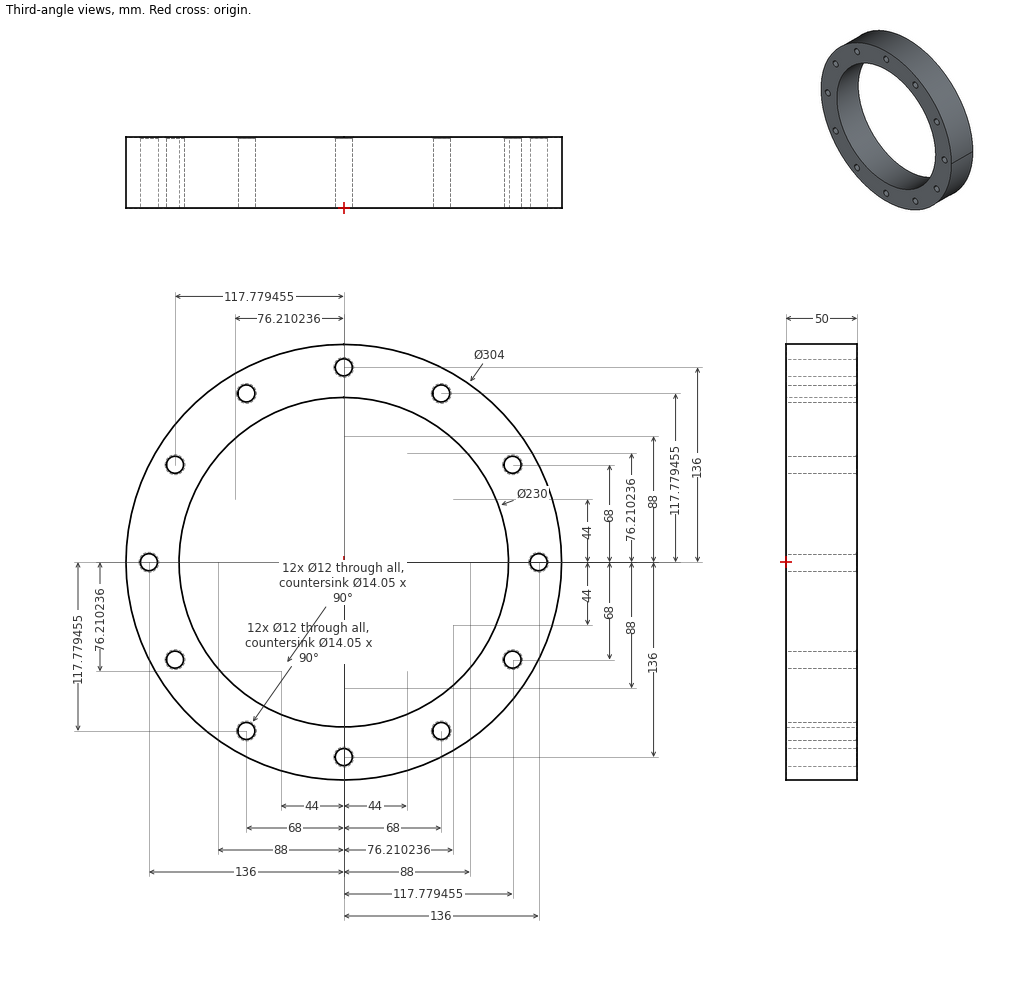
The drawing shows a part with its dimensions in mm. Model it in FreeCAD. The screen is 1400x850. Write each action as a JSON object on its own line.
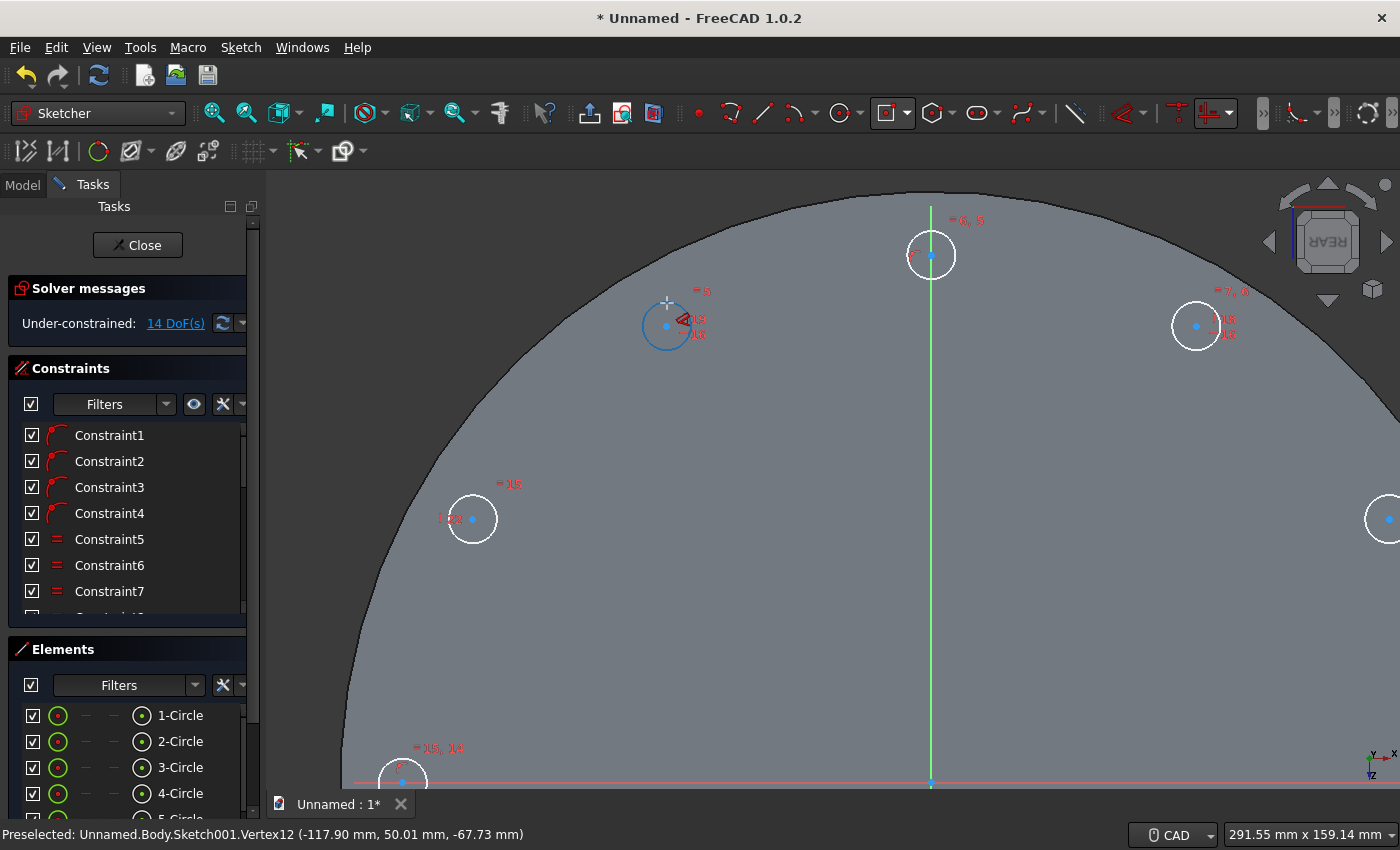
{"action": "left_click", "coordinate": [668, 302]}
{"action": "left_click", "coordinate": [669, 270]}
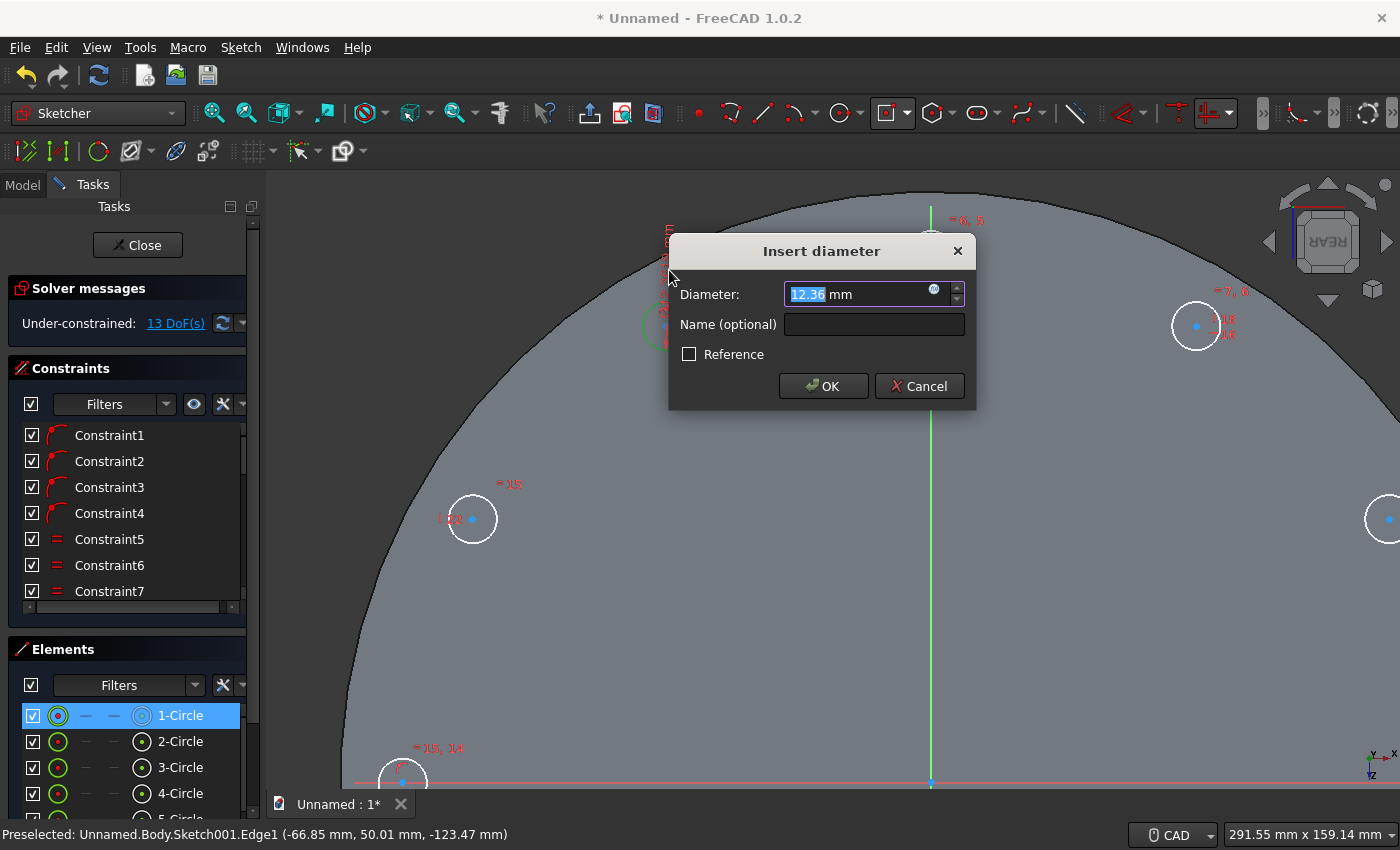
{"action": "type", "text": "12"}
{"action": "key", "text": "Return"}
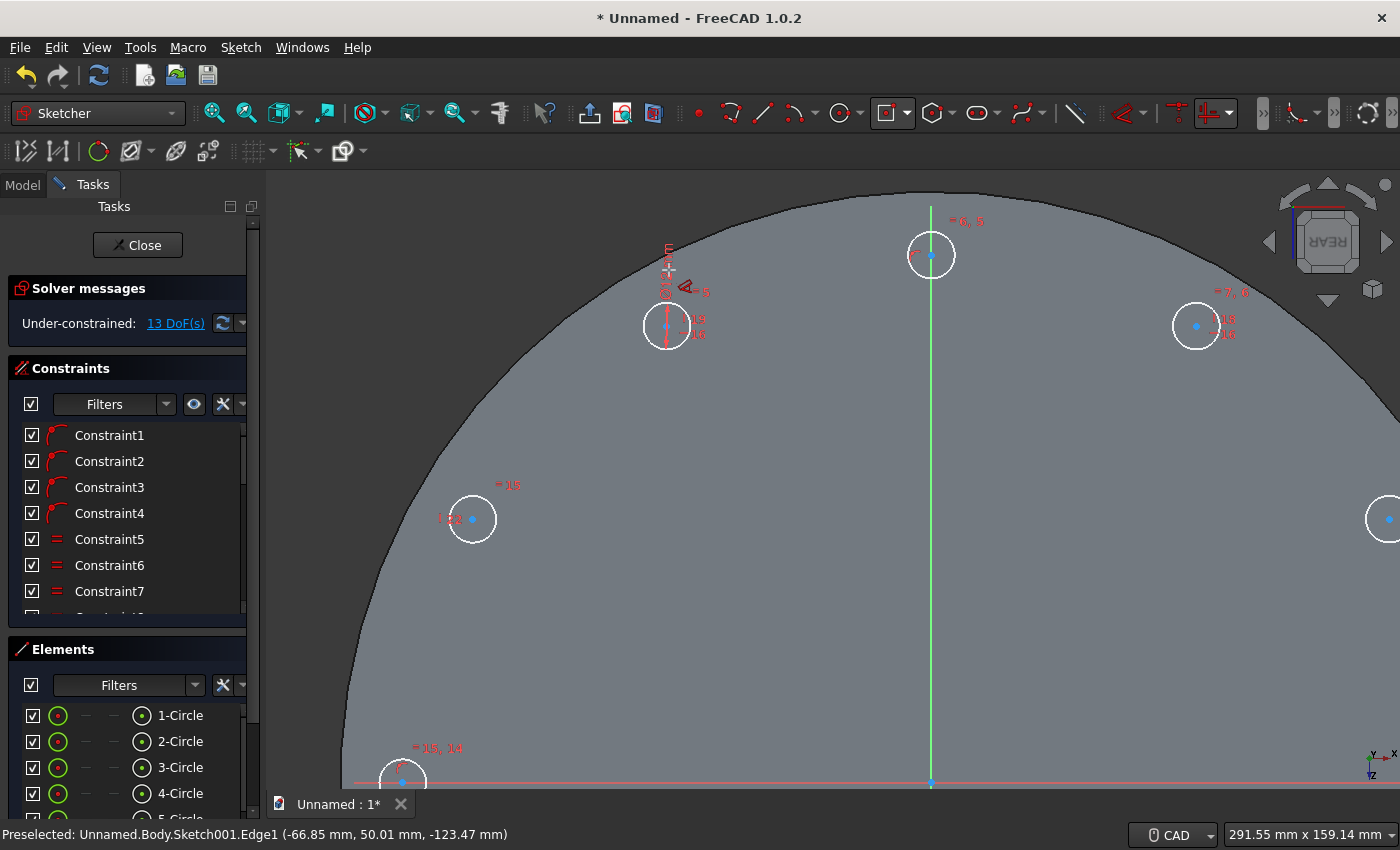
{"action": "left_click", "coordinate": [667, 326]}
{"action": "left_click", "coordinate": [799, 292]}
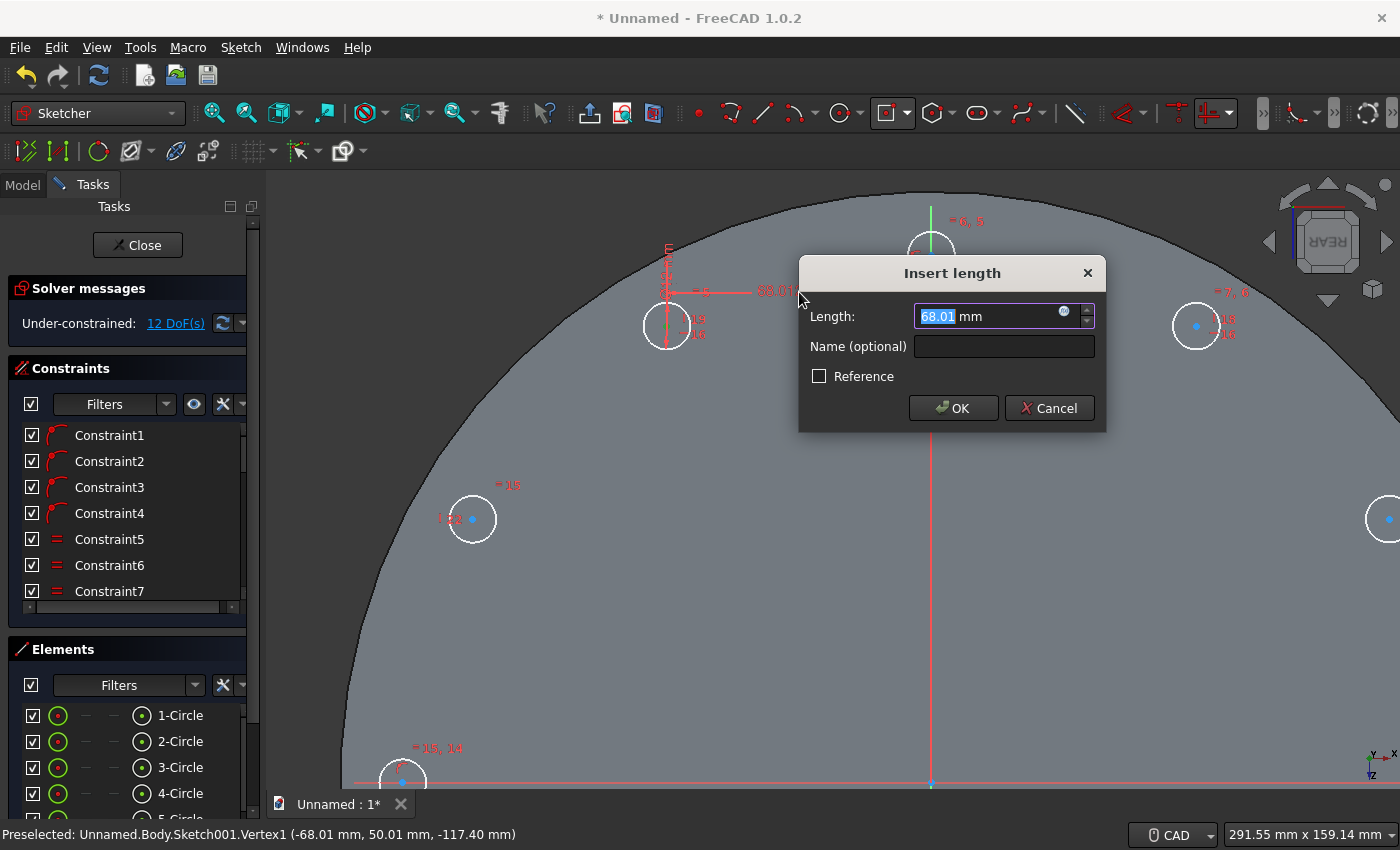
{"action": "type", "text": "68"}
{"action": "key", "text": "Return"}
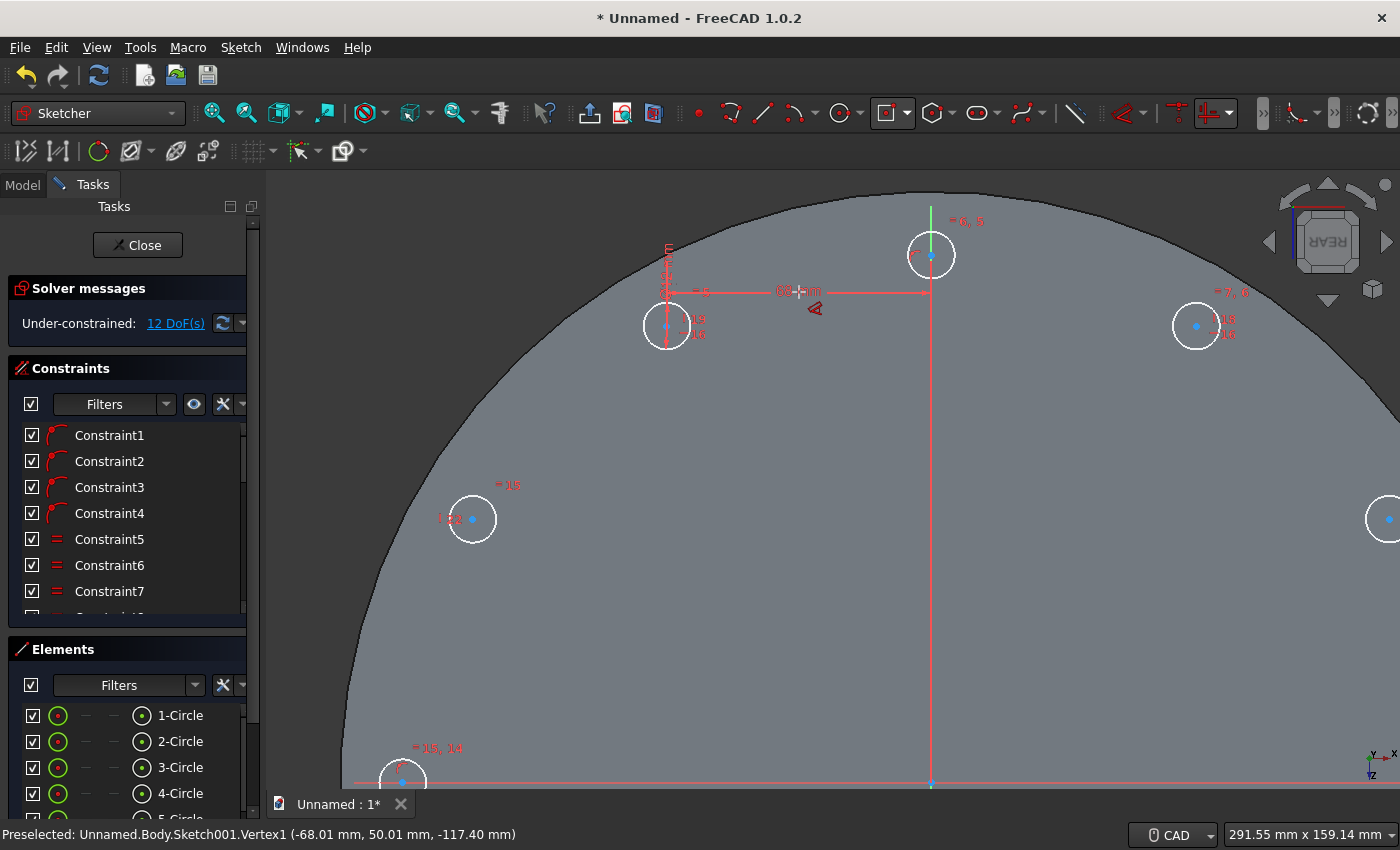
{"action": "left_click", "coordinate": [1196, 326]}
{"action": "left_click", "coordinate": [1064, 292]}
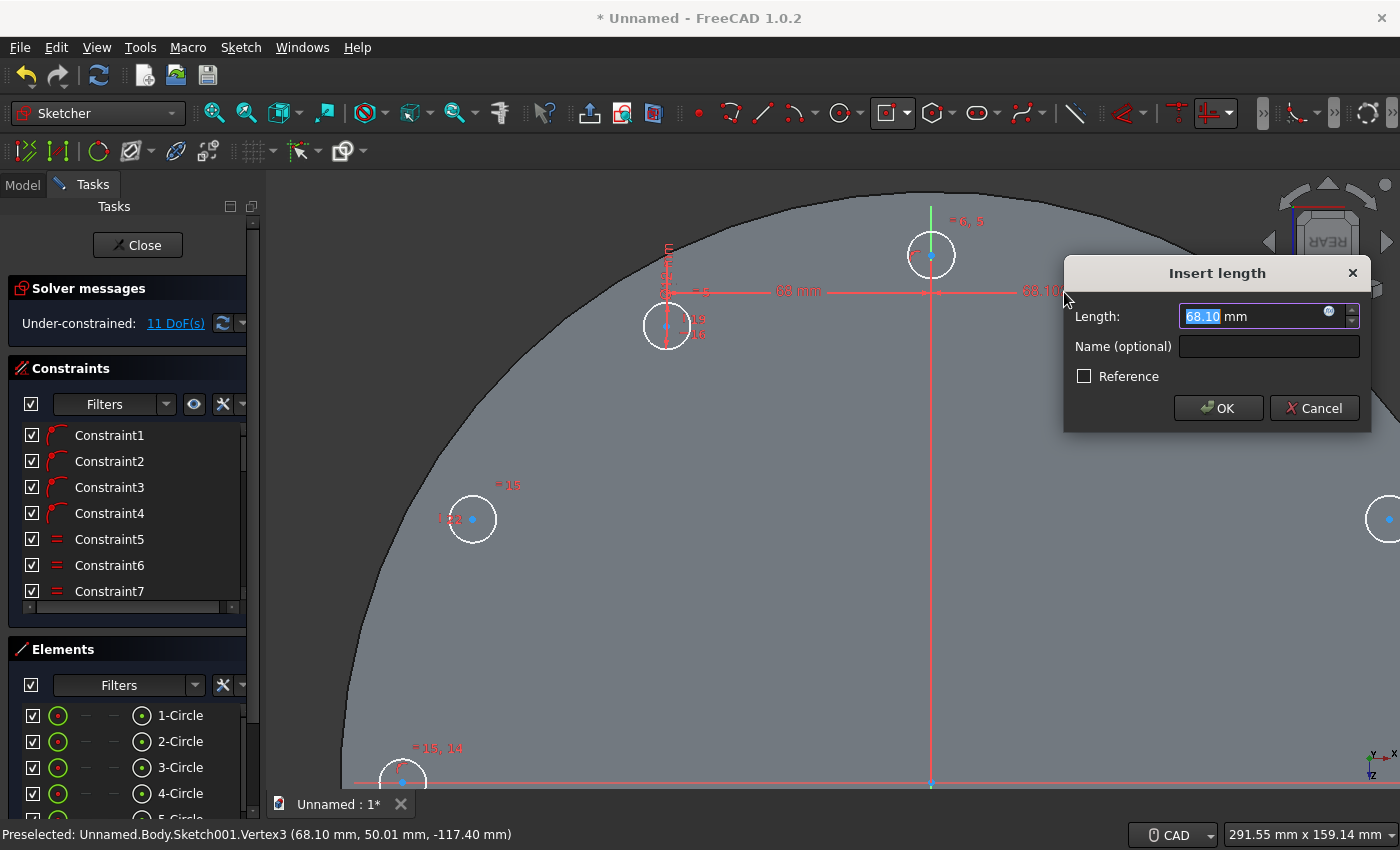
{"action": "type", "text": "68"}
{"action": "key", "text": "Return"}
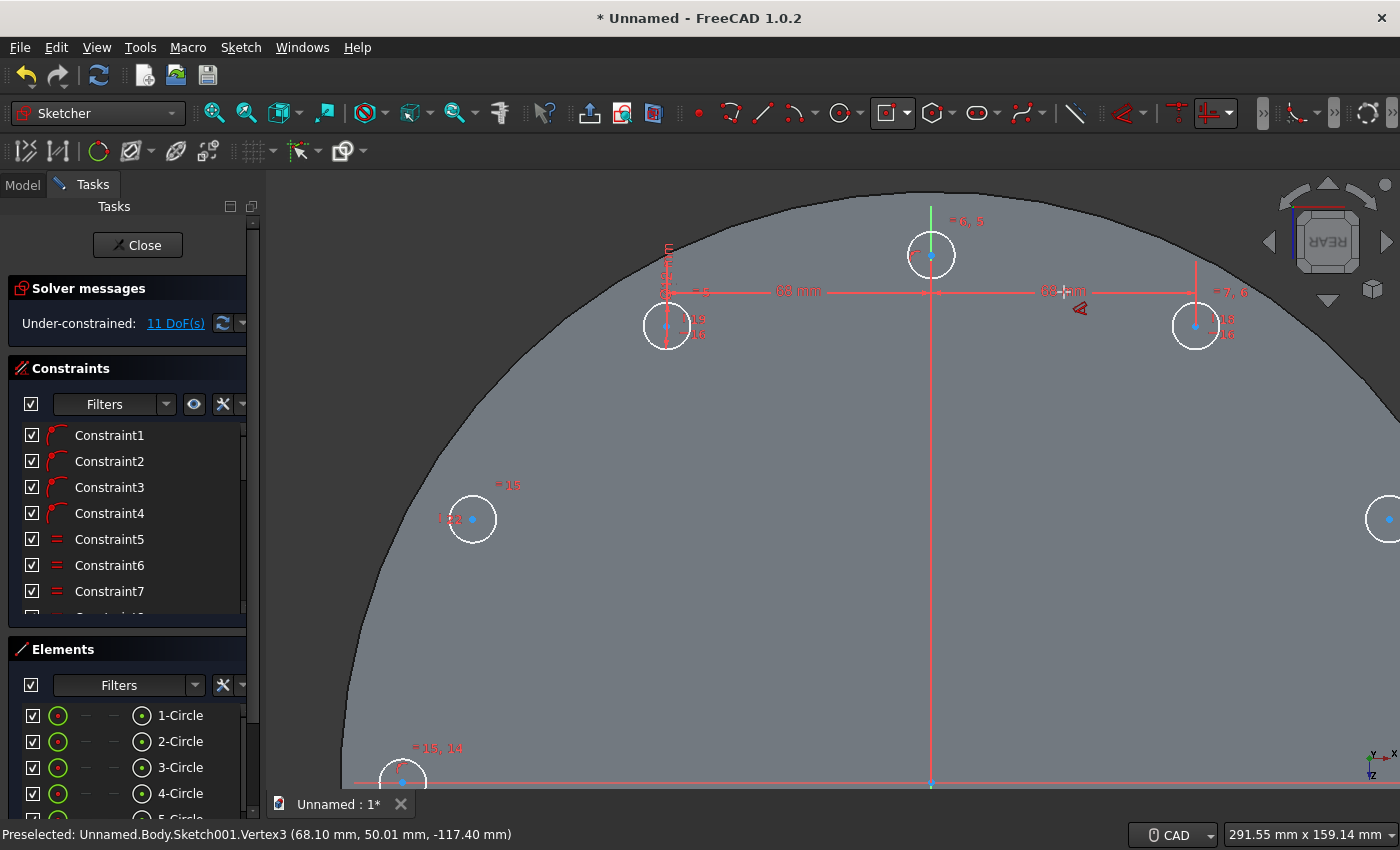
{"action": "scroll", "coordinate": [667, 303], "scroll_direction": "down", "scroll_amount": 5}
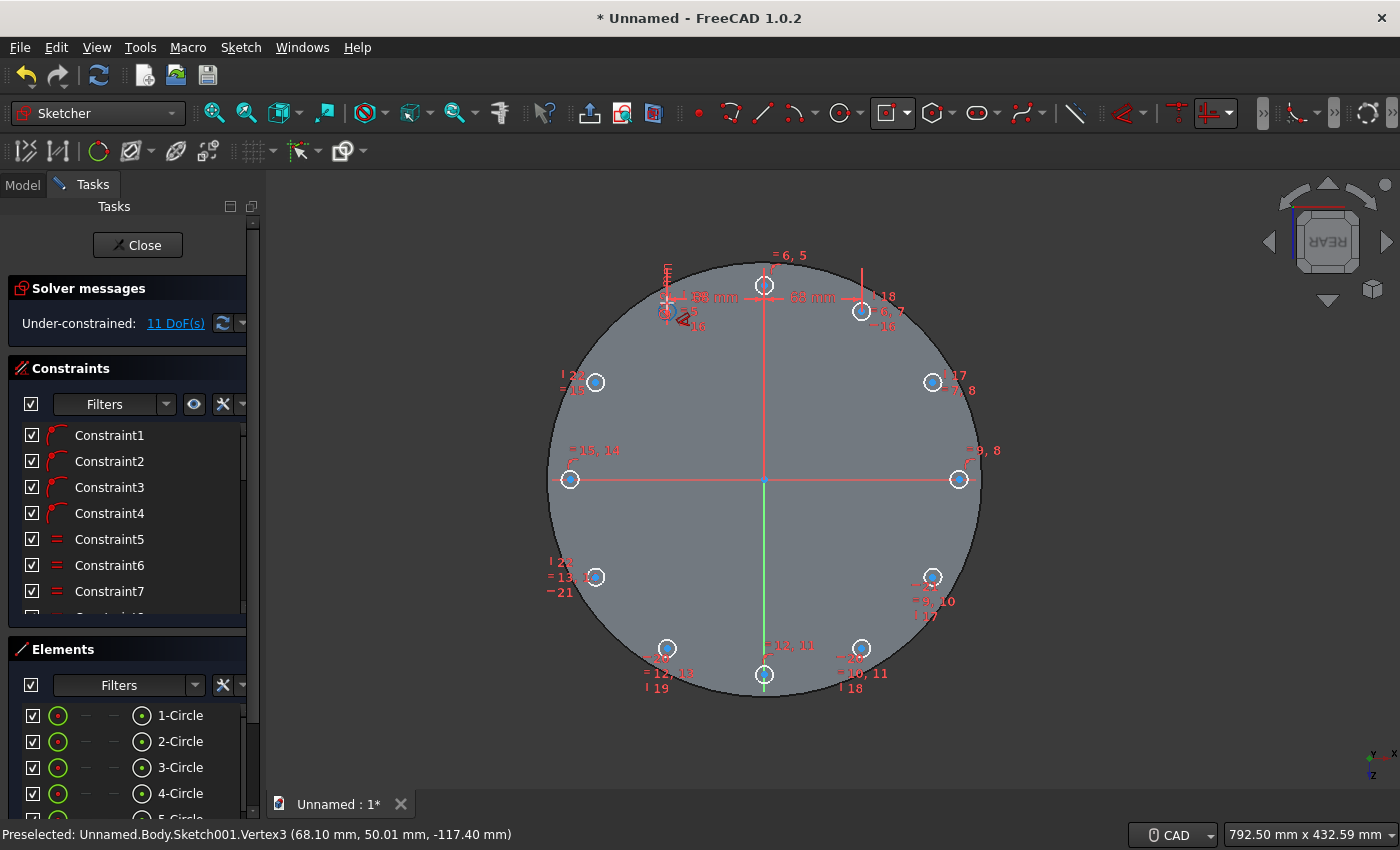
{"action": "left_click", "coordinate": [933, 383]}
{"action": "left_click", "coordinate": [967, 431]}